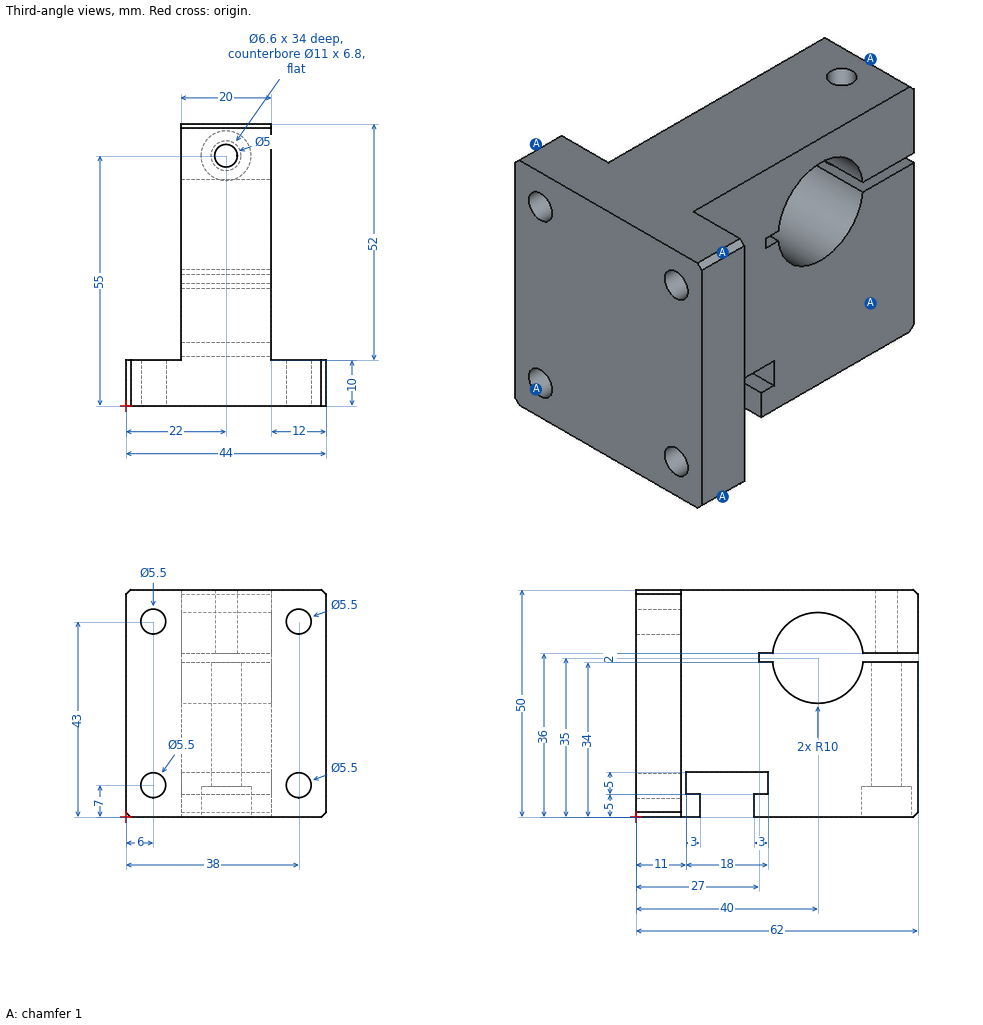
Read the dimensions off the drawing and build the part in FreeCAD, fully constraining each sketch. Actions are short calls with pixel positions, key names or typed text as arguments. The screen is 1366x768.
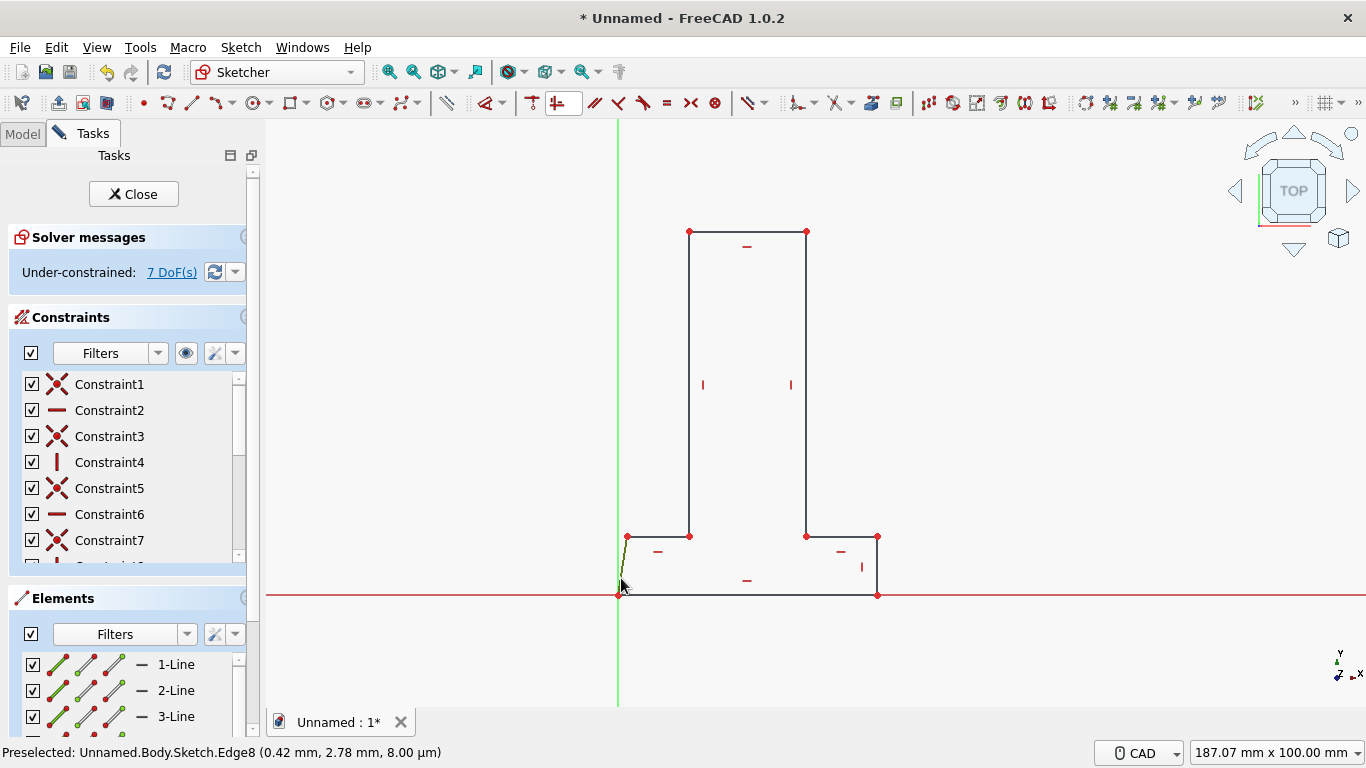
click(576, 104)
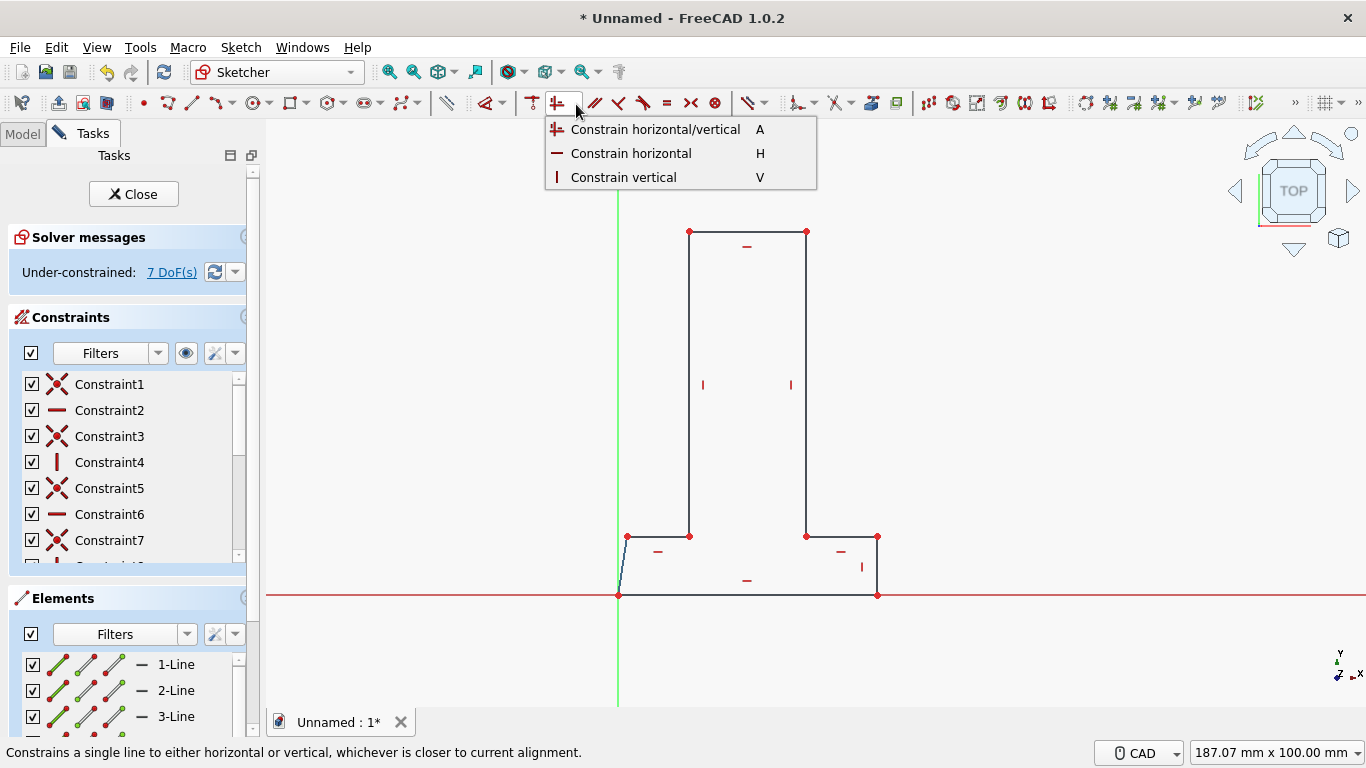
click(681, 177)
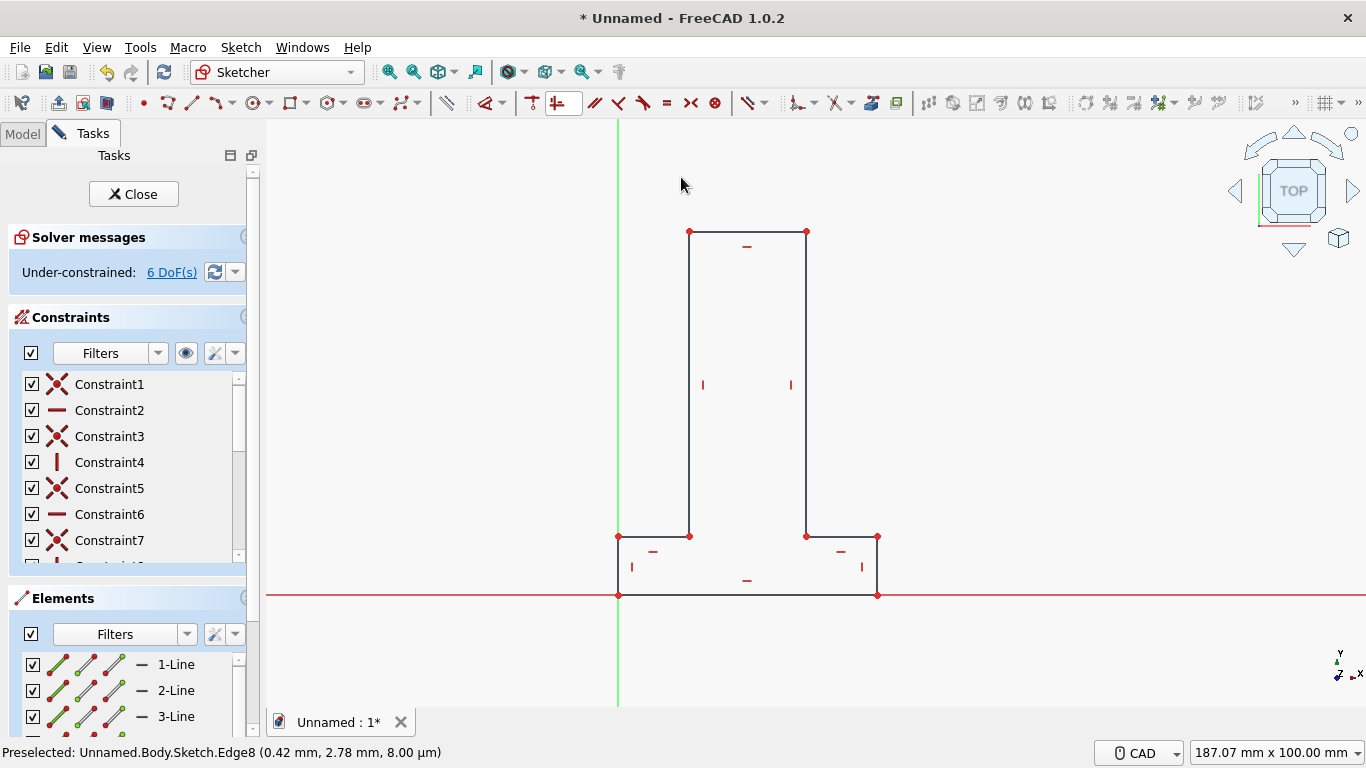
click(486, 104)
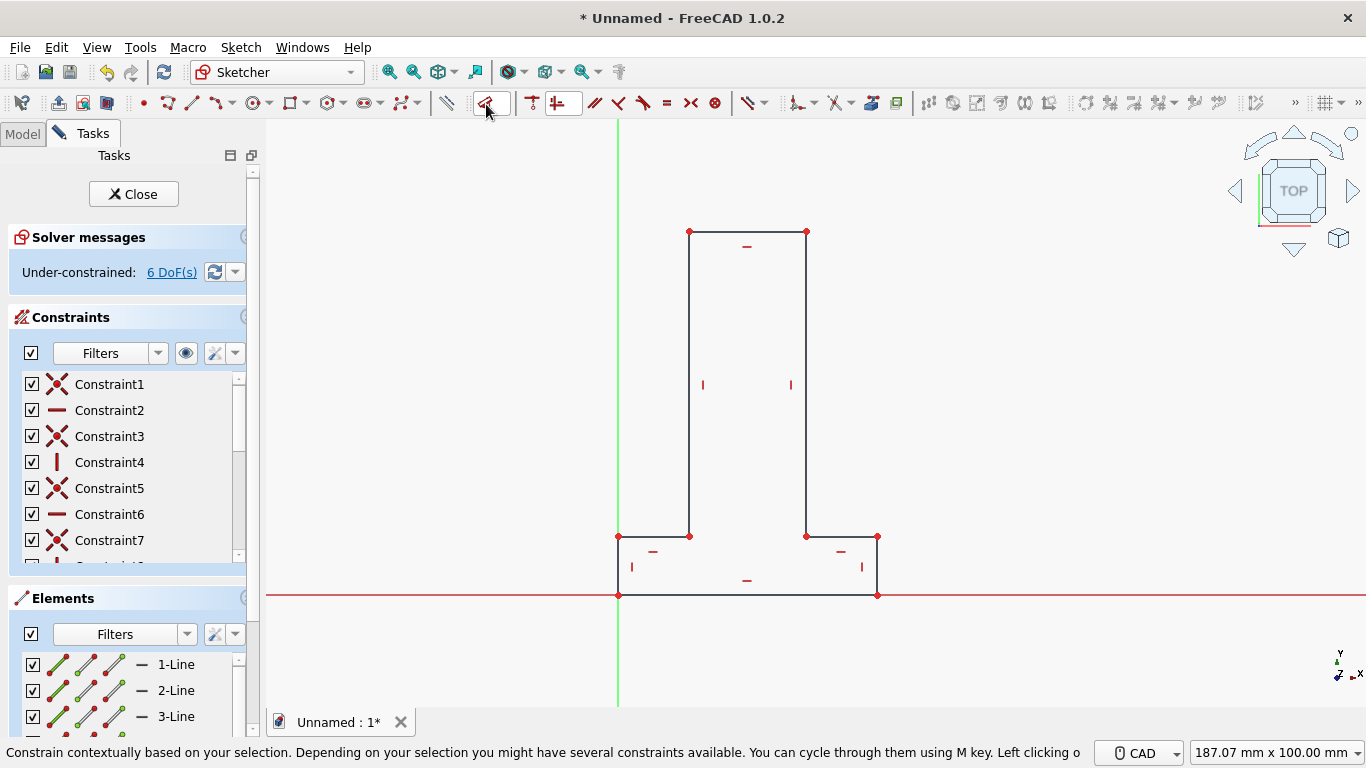
click(696, 595)
click(748, 629)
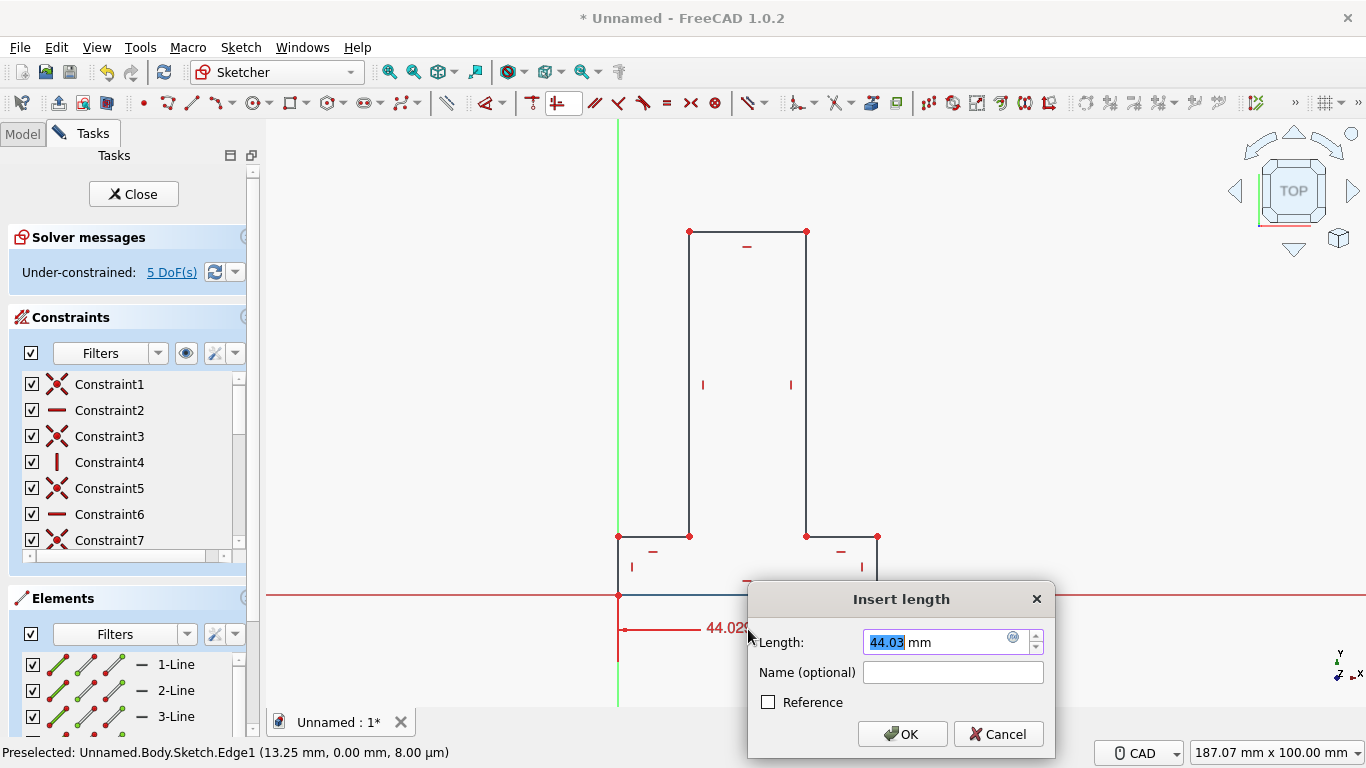
text(44)
key(Return)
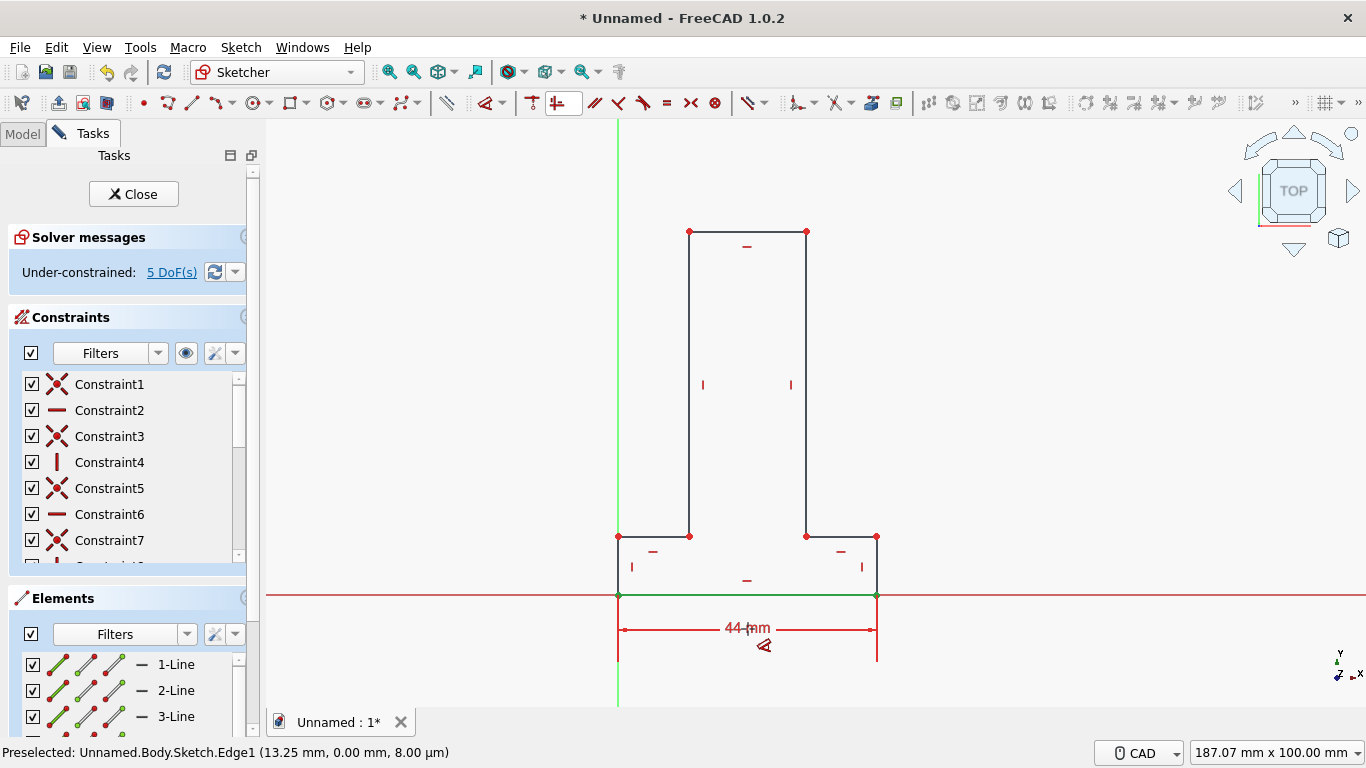
click(877, 578)
click(911, 566)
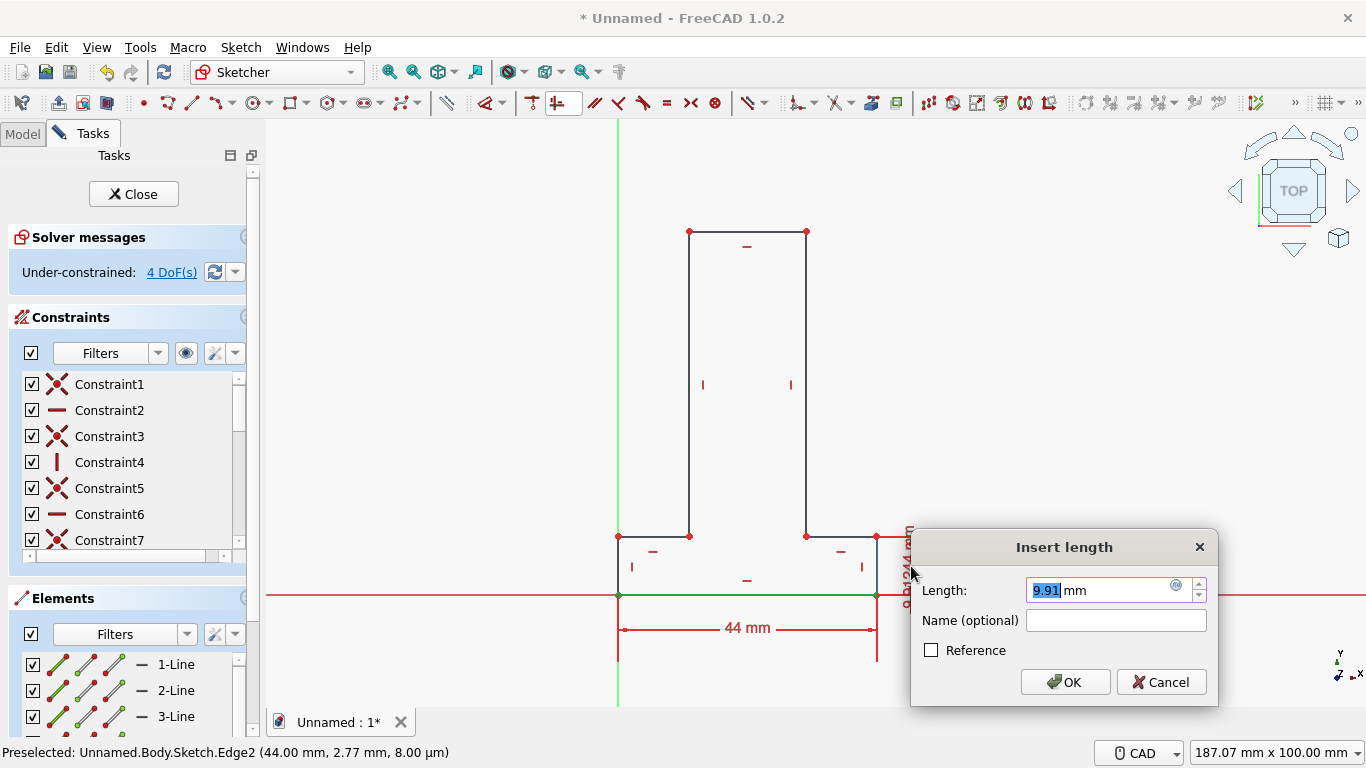
text(10)
key(Return)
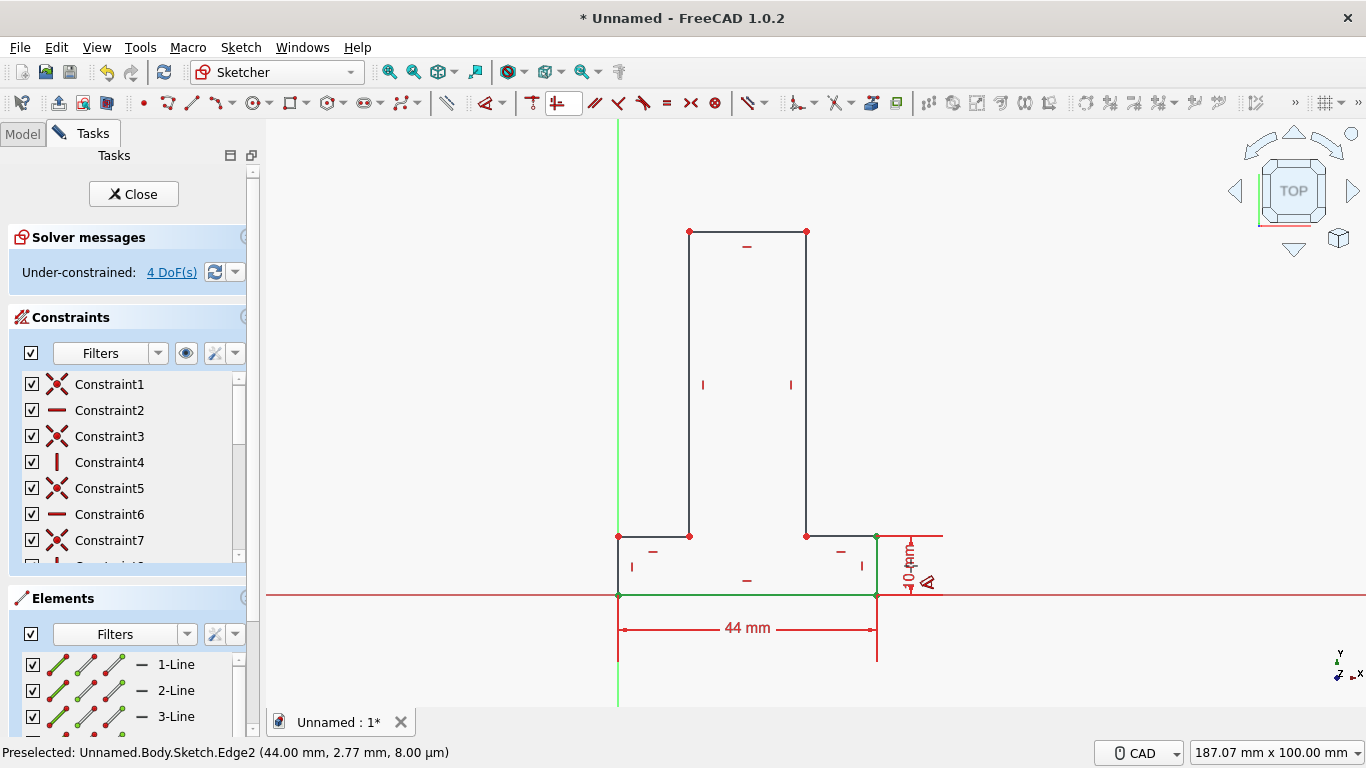
click(856, 536)
click(825, 570)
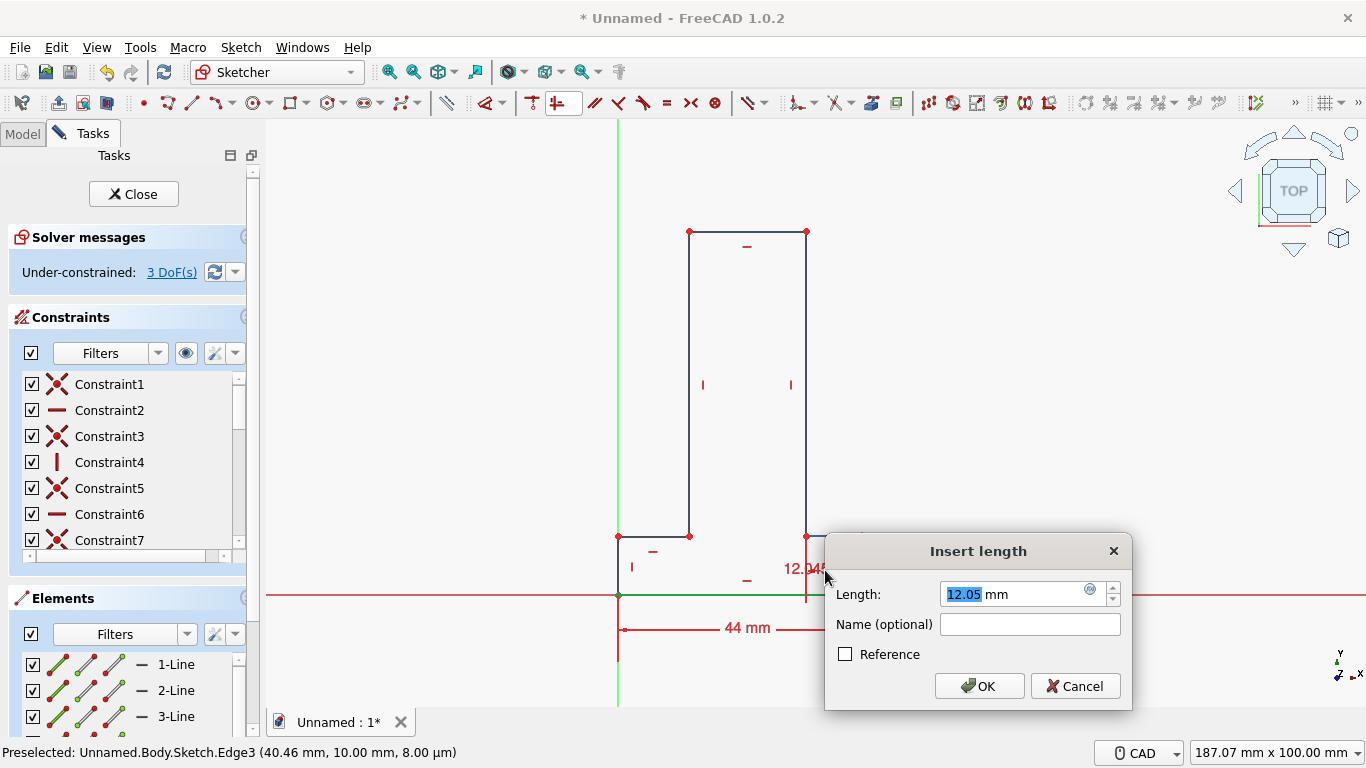
text(12)
key(Return)